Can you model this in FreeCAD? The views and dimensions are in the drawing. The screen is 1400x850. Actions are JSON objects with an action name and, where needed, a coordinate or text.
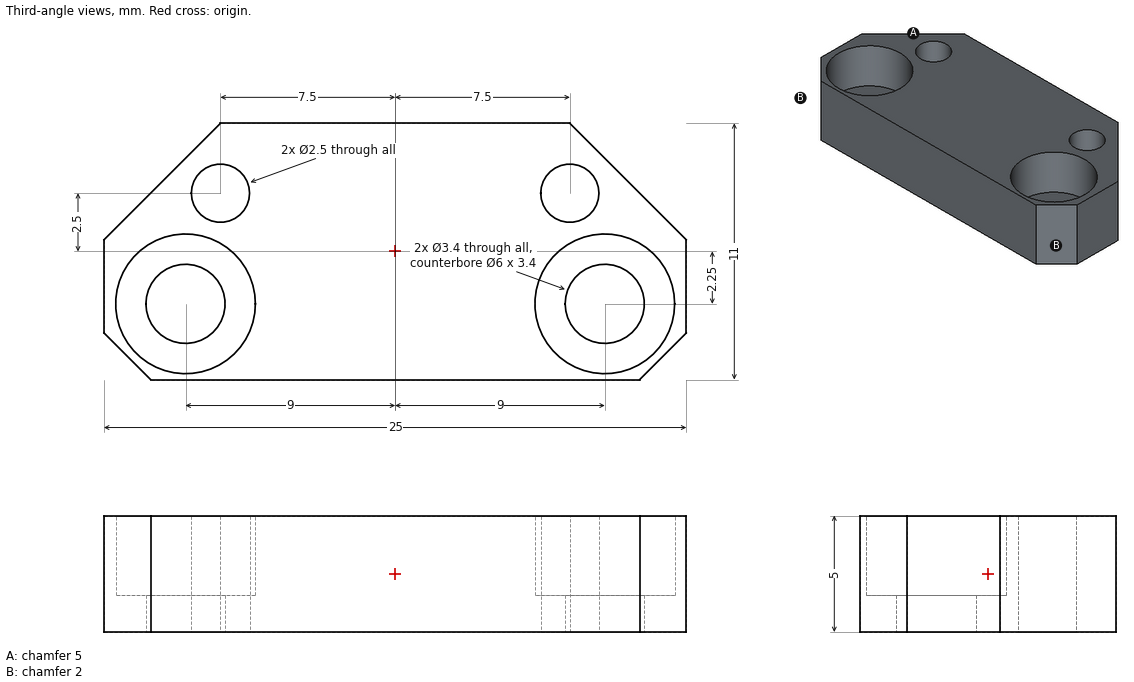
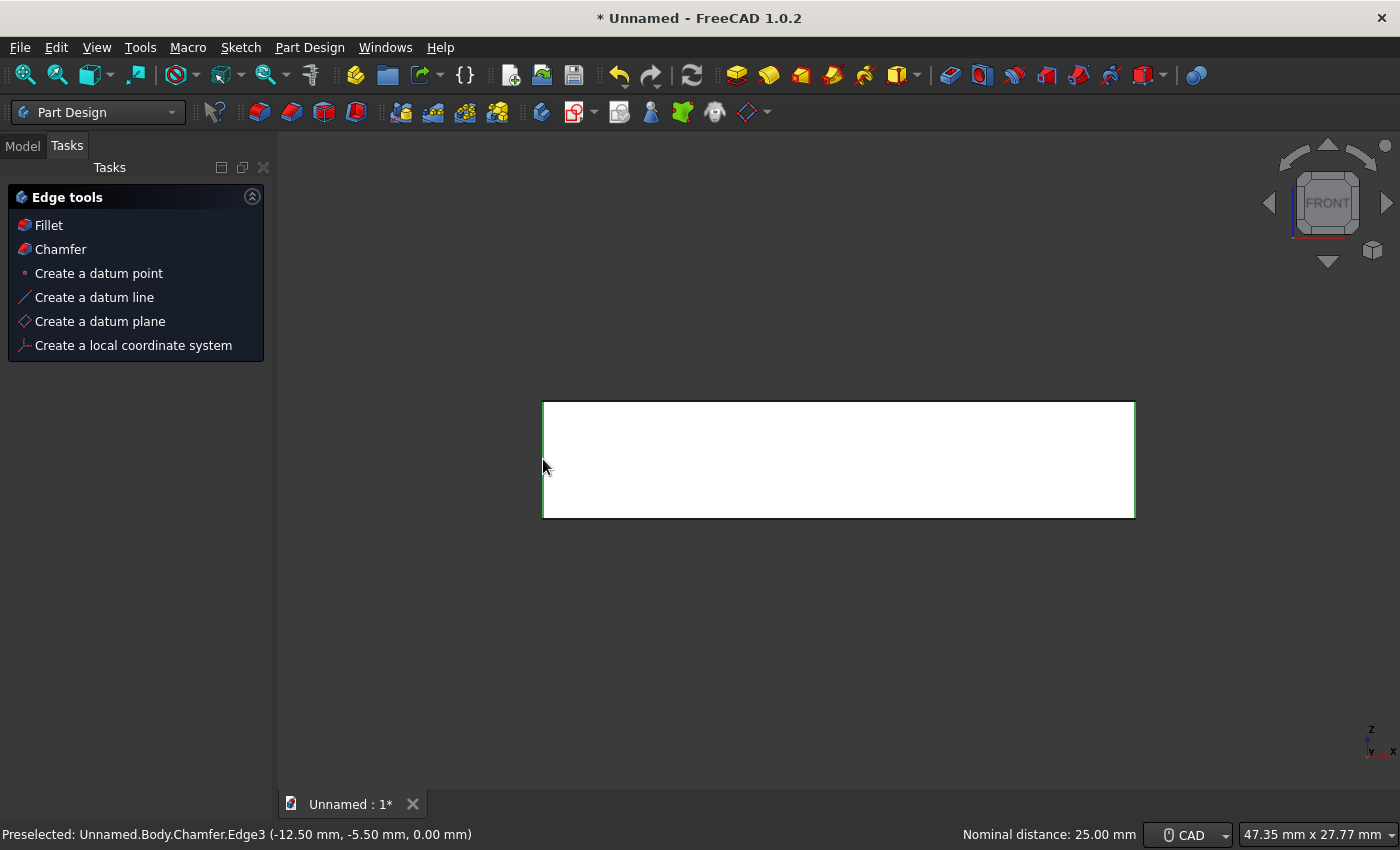
{"action": "left_click", "coordinate": [292, 112]}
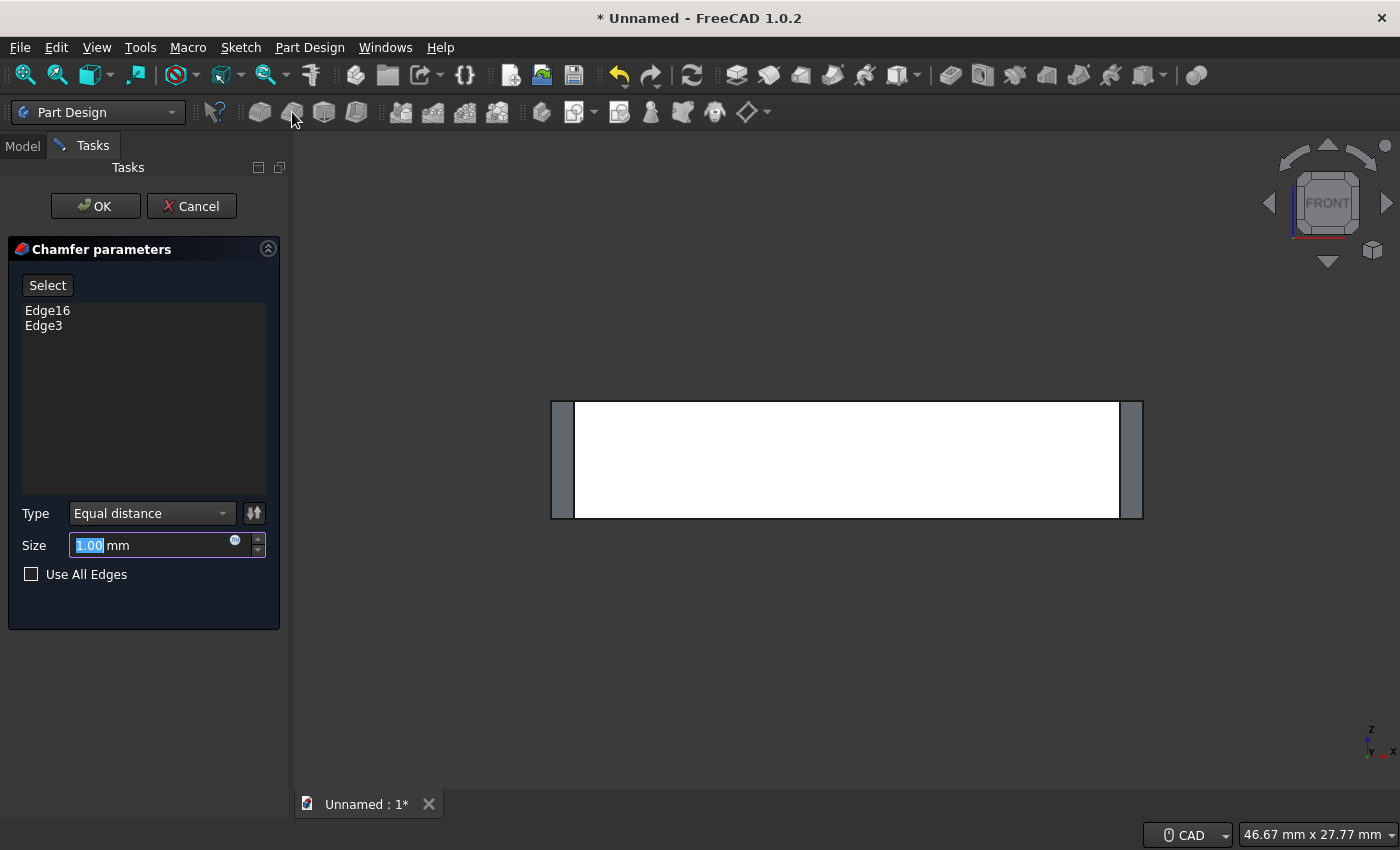
{"action": "type", "text": "2"}
{"action": "key", "text": "Tab"}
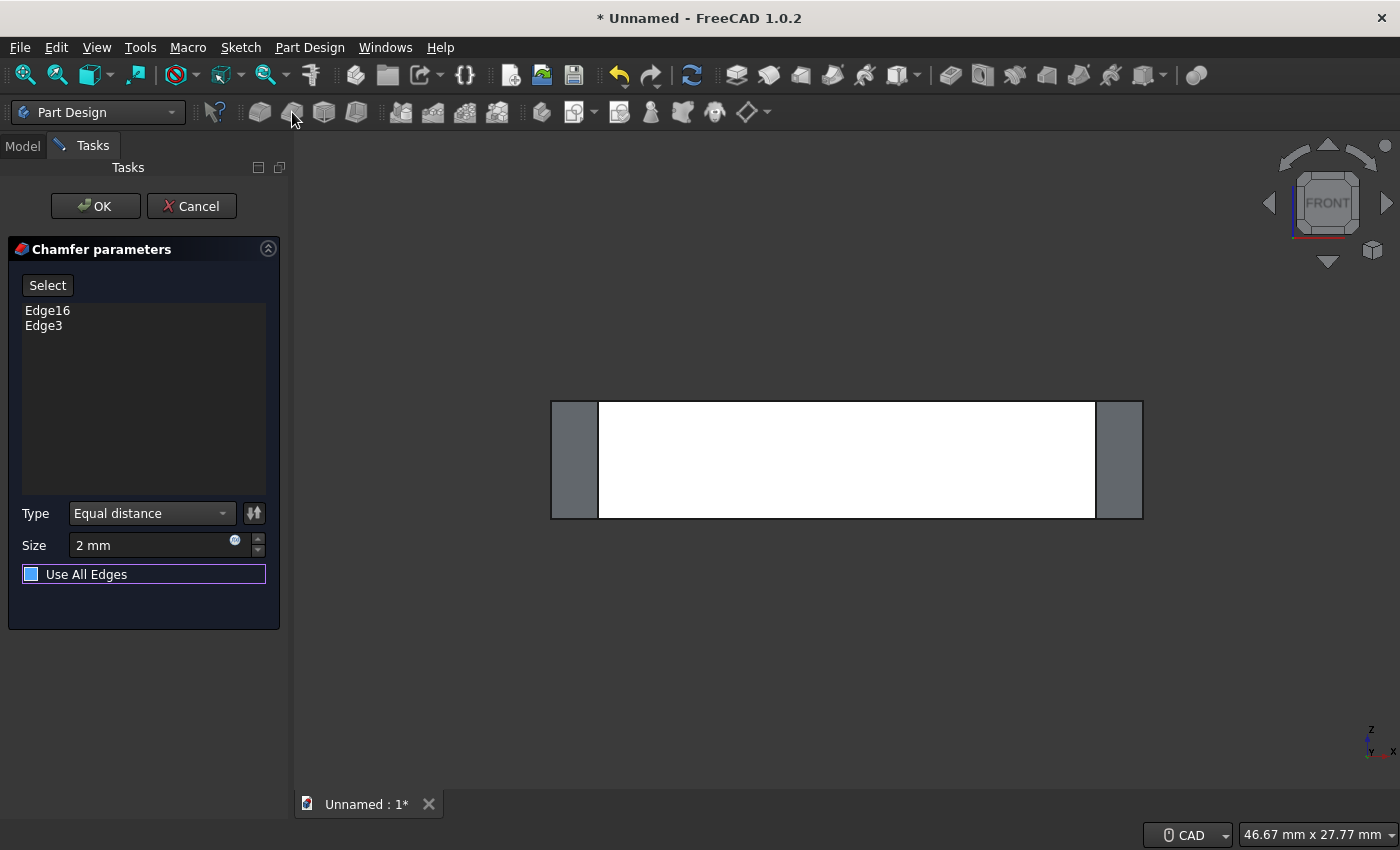
{"action": "left_click", "coordinate": [96, 206]}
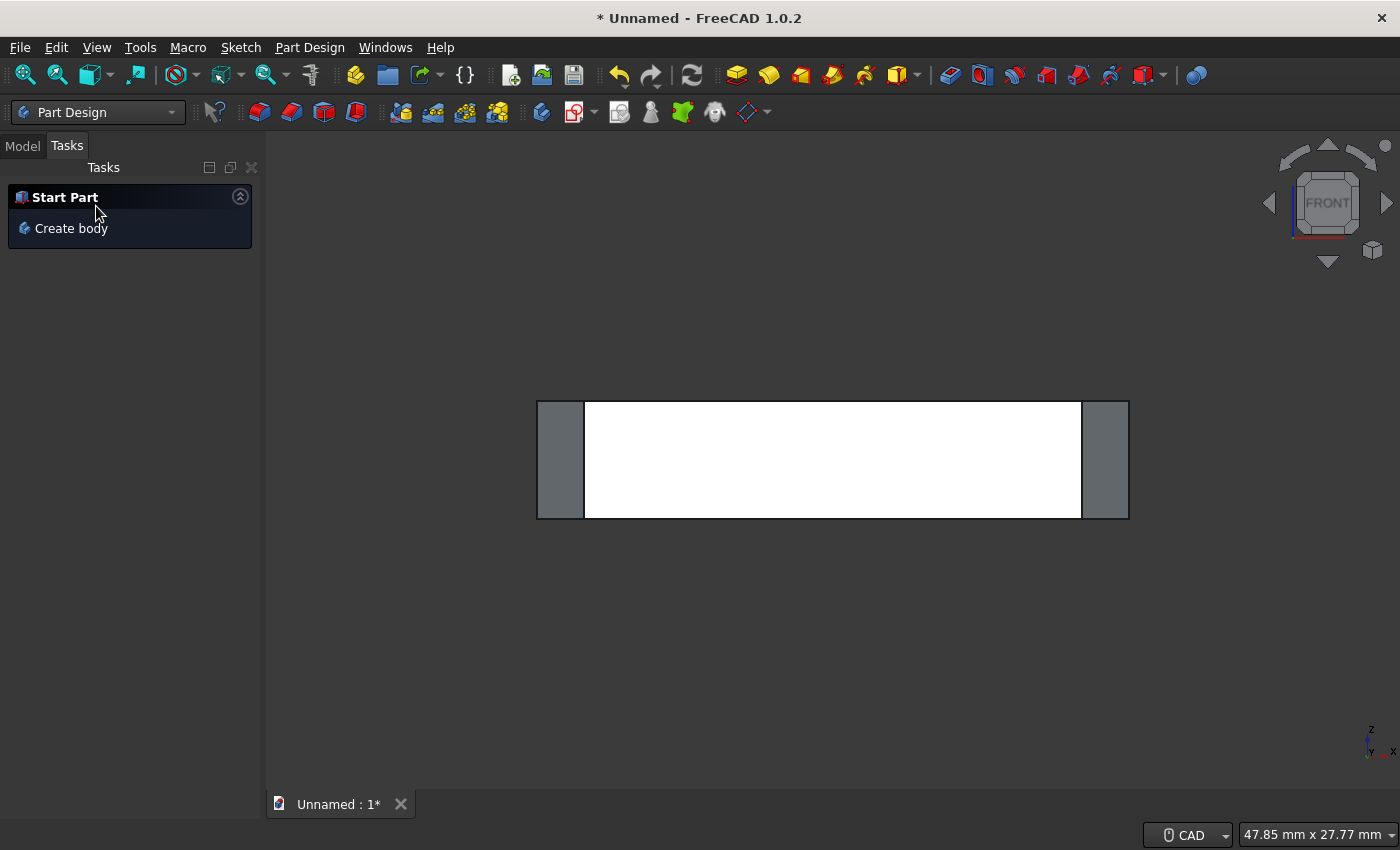
{"action": "key", "text": "0"}